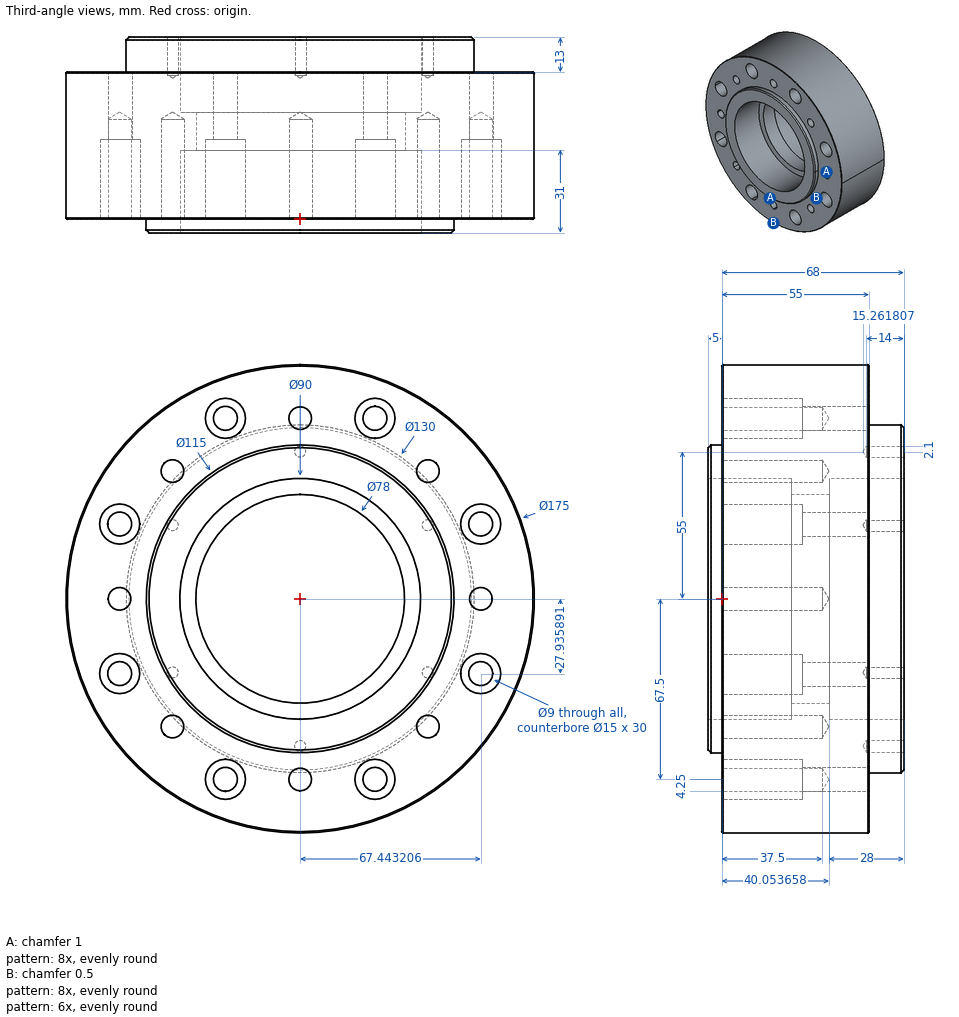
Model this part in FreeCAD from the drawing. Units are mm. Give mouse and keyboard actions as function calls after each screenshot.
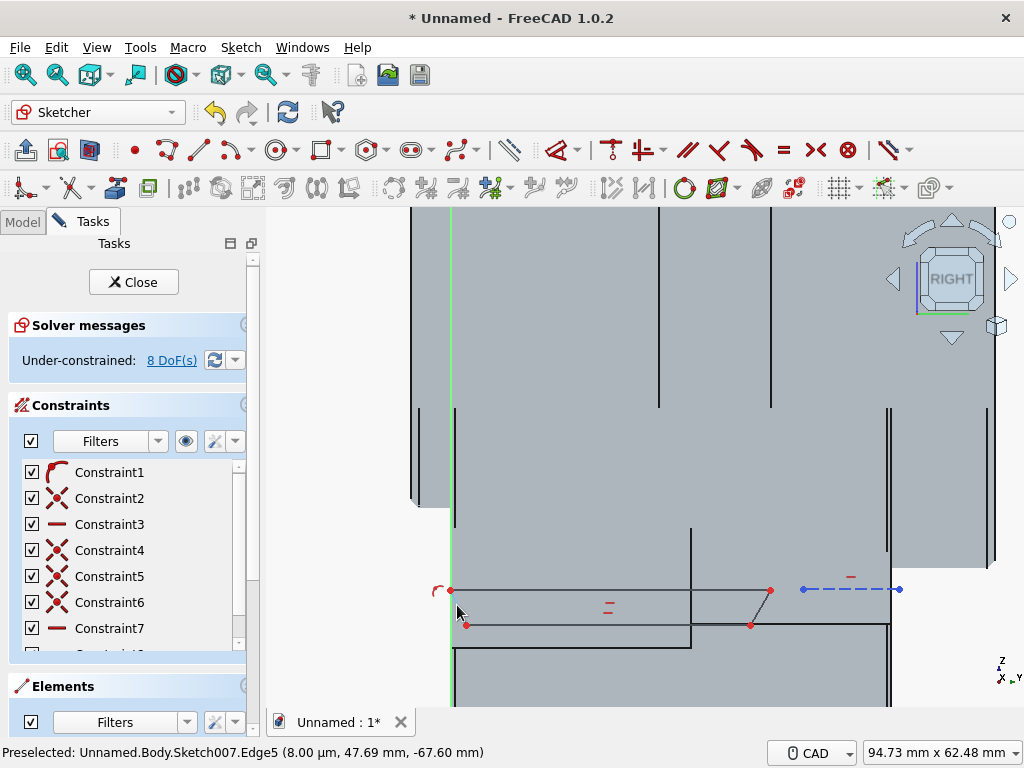
click(457, 604)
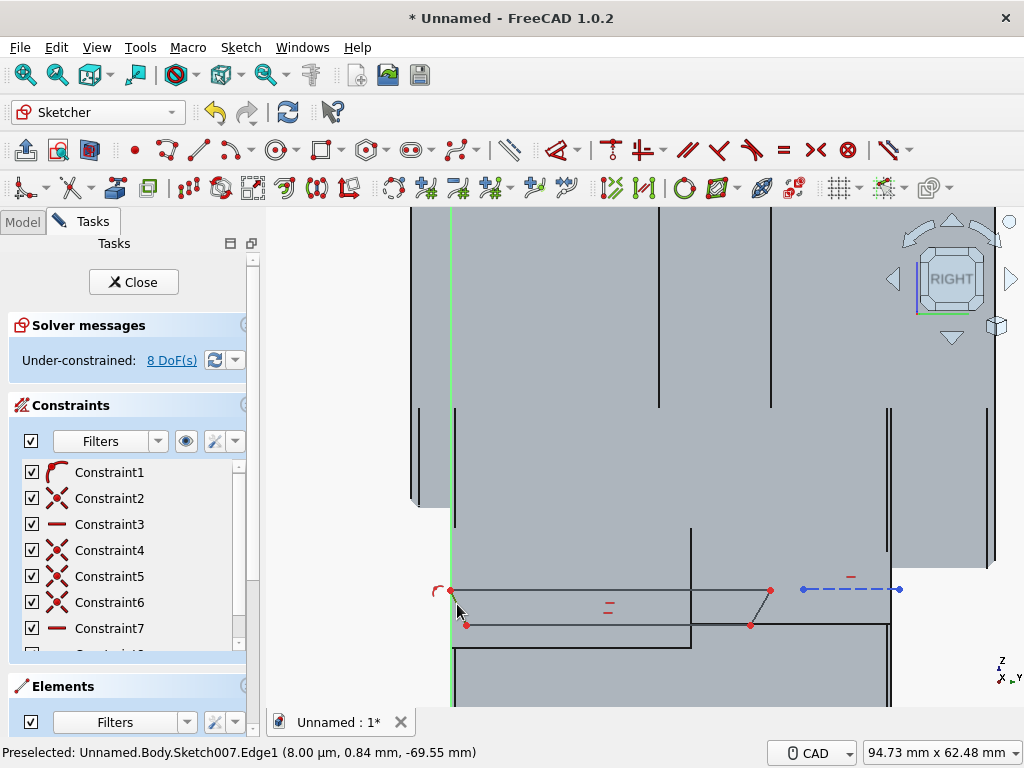
click(666, 150)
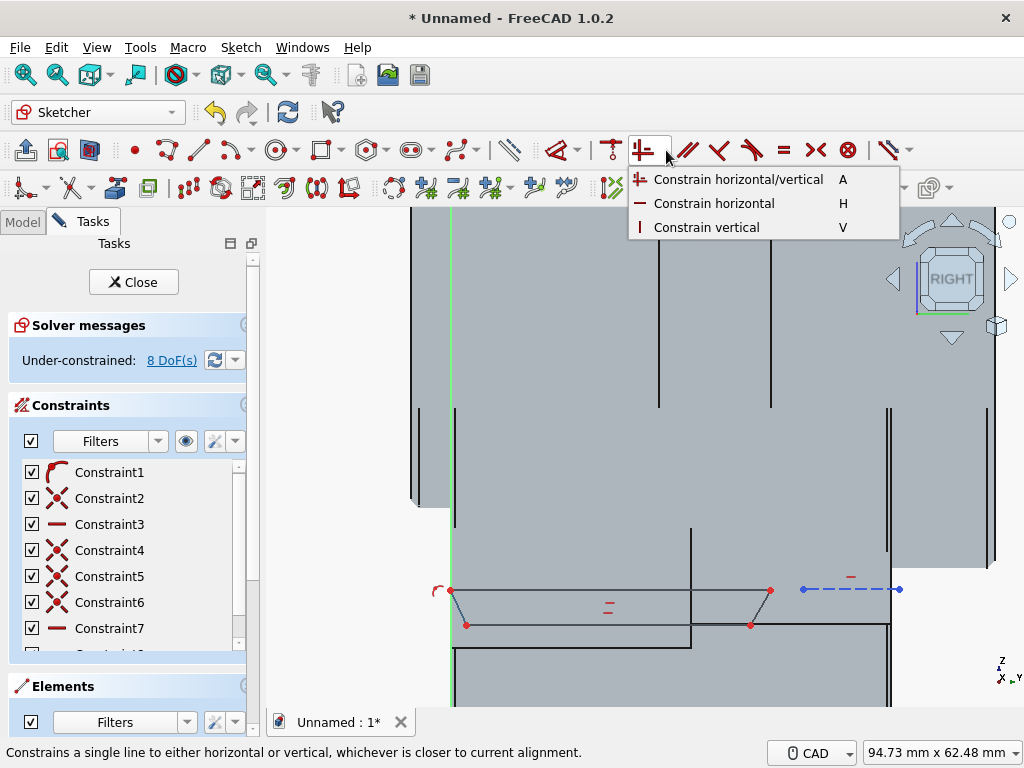
click(764, 227)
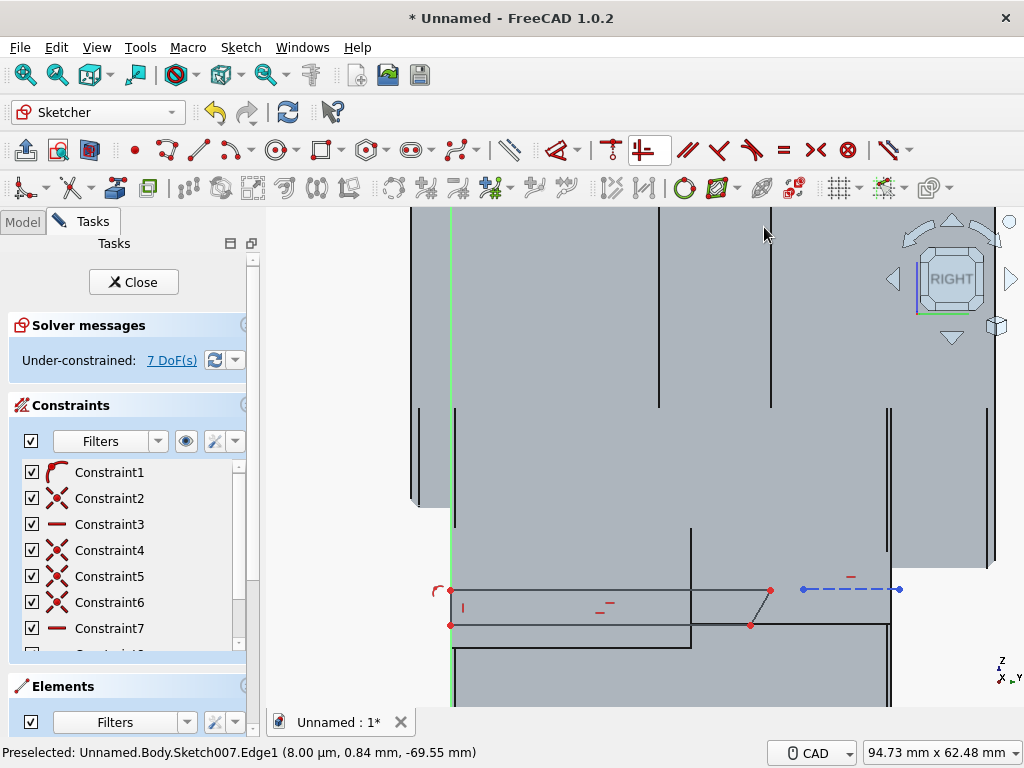
click(556, 150)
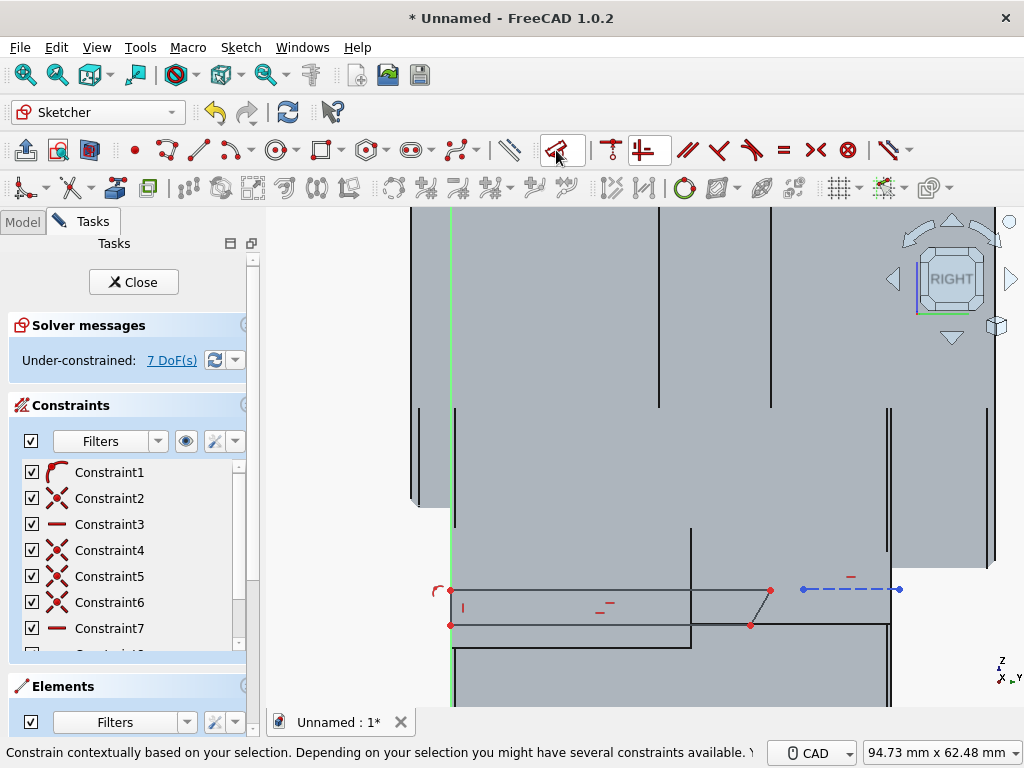
scroll(451, 601, up, 2)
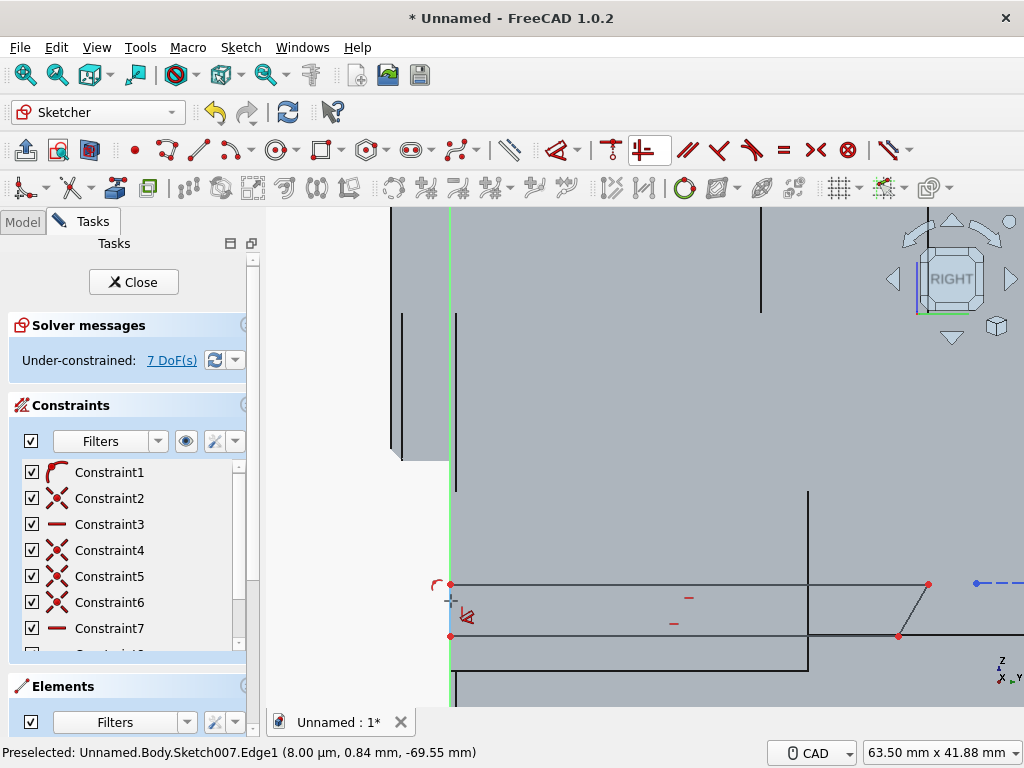
click(450, 600)
click(416, 611)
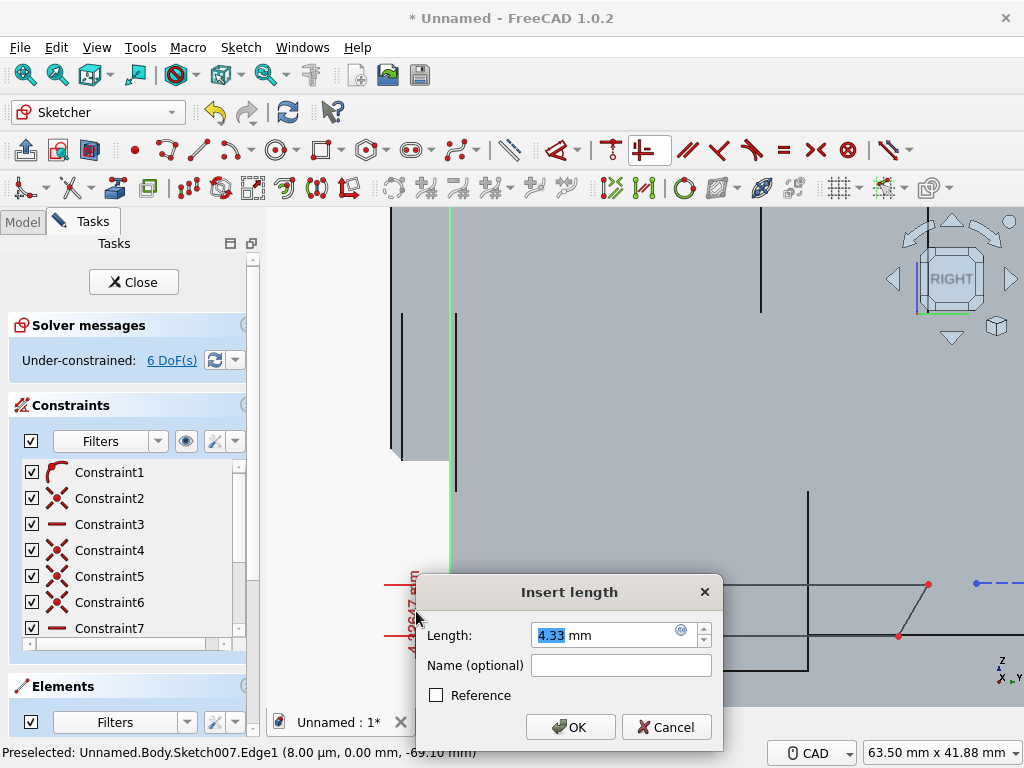
text(4.25)
key(Return)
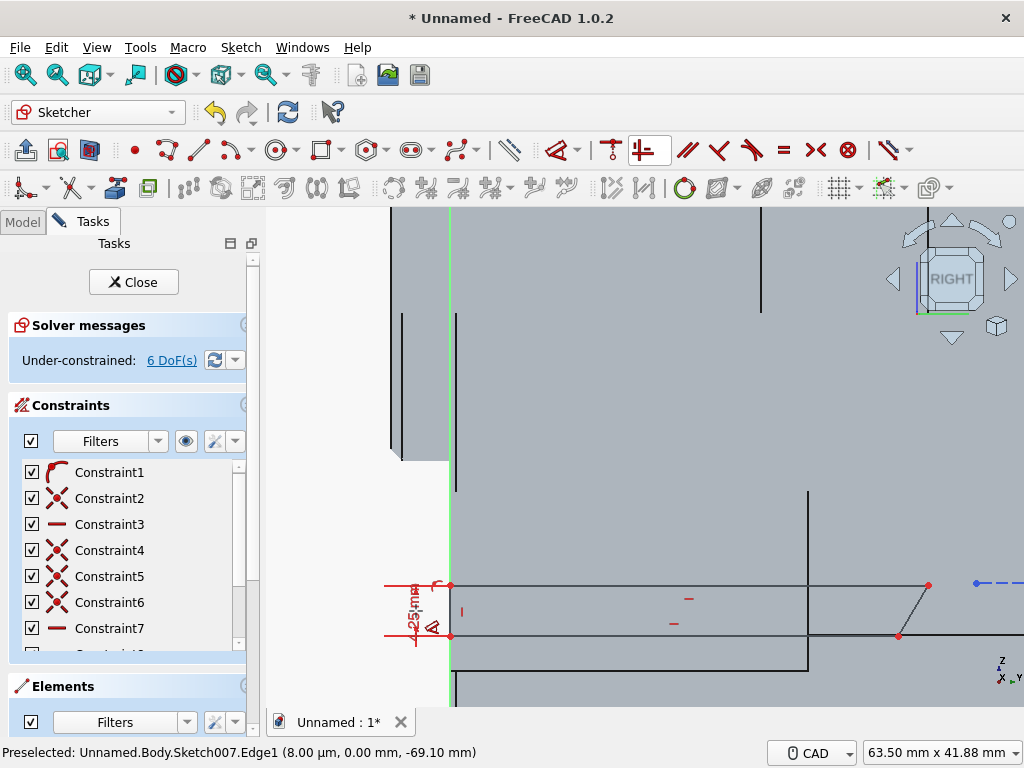
click(585, 636)
click(655, 670)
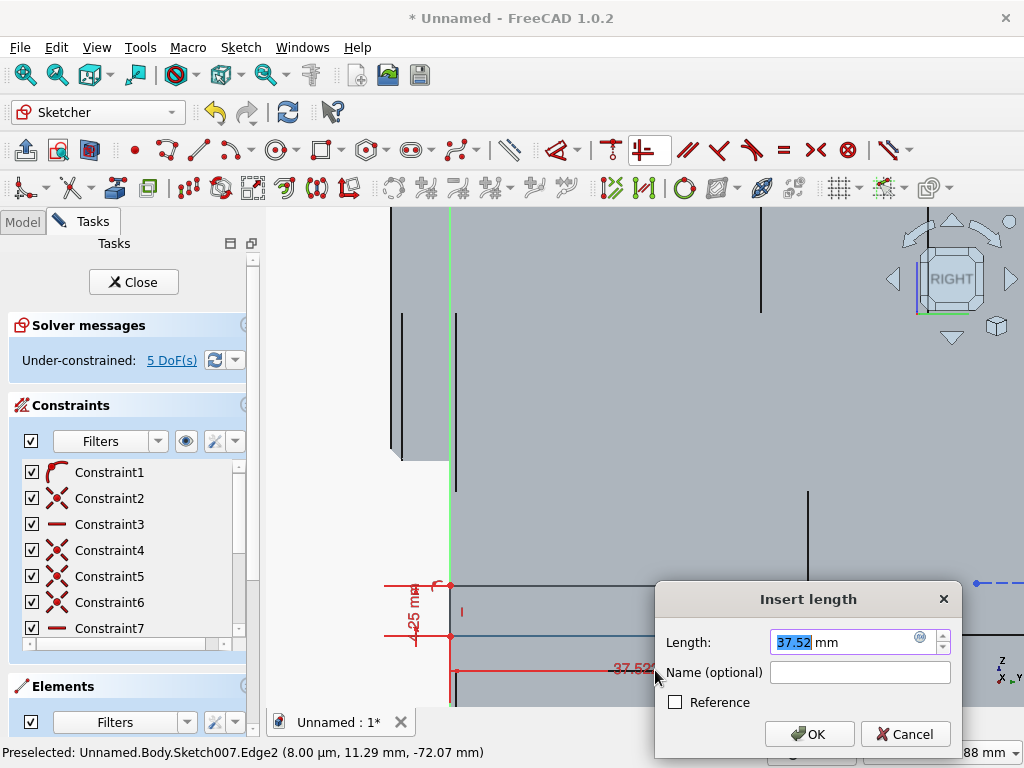
text(37.5)
key(Return)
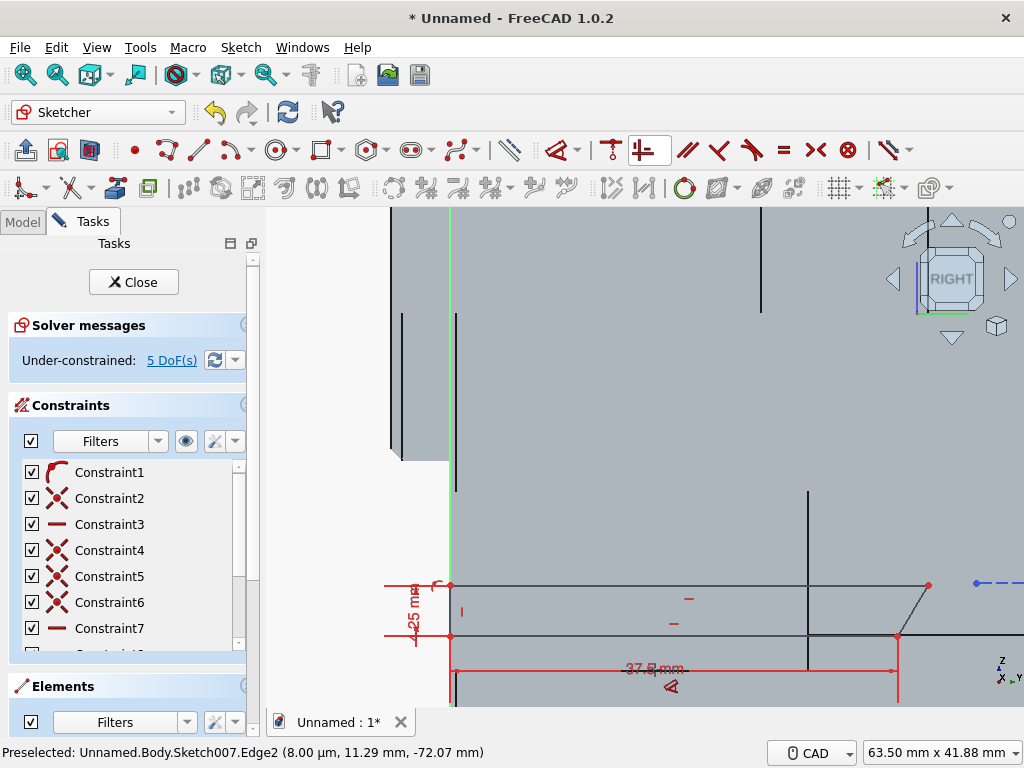
click(450, 586)
click(416, 410)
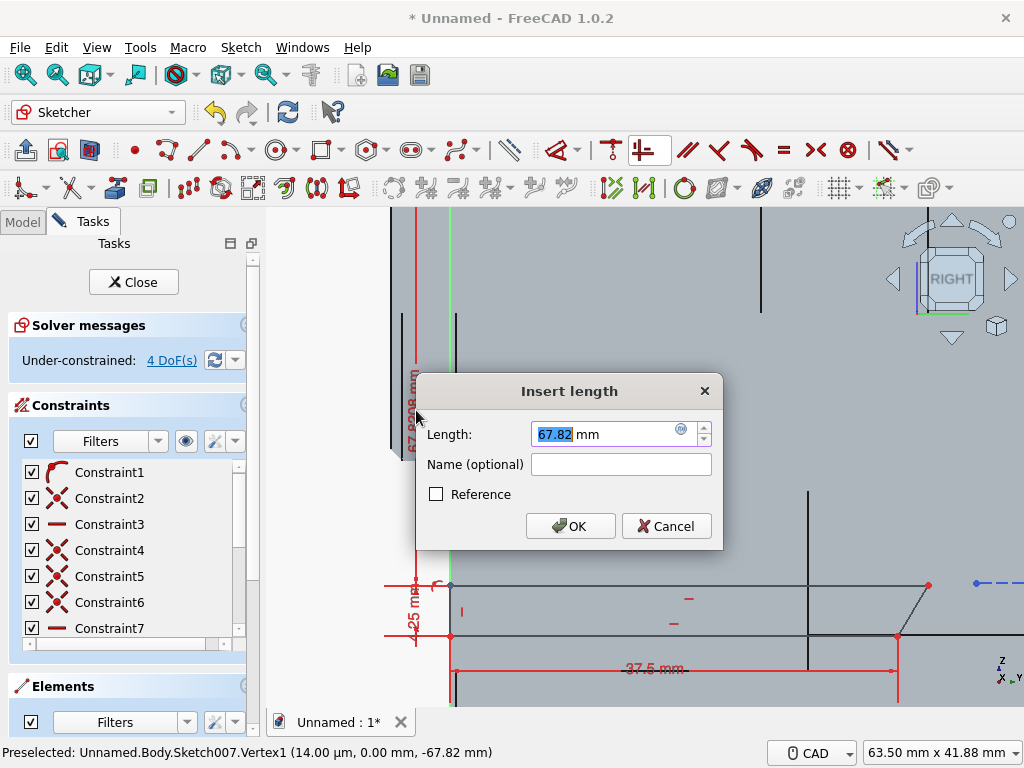
text(67.5)
key(Return)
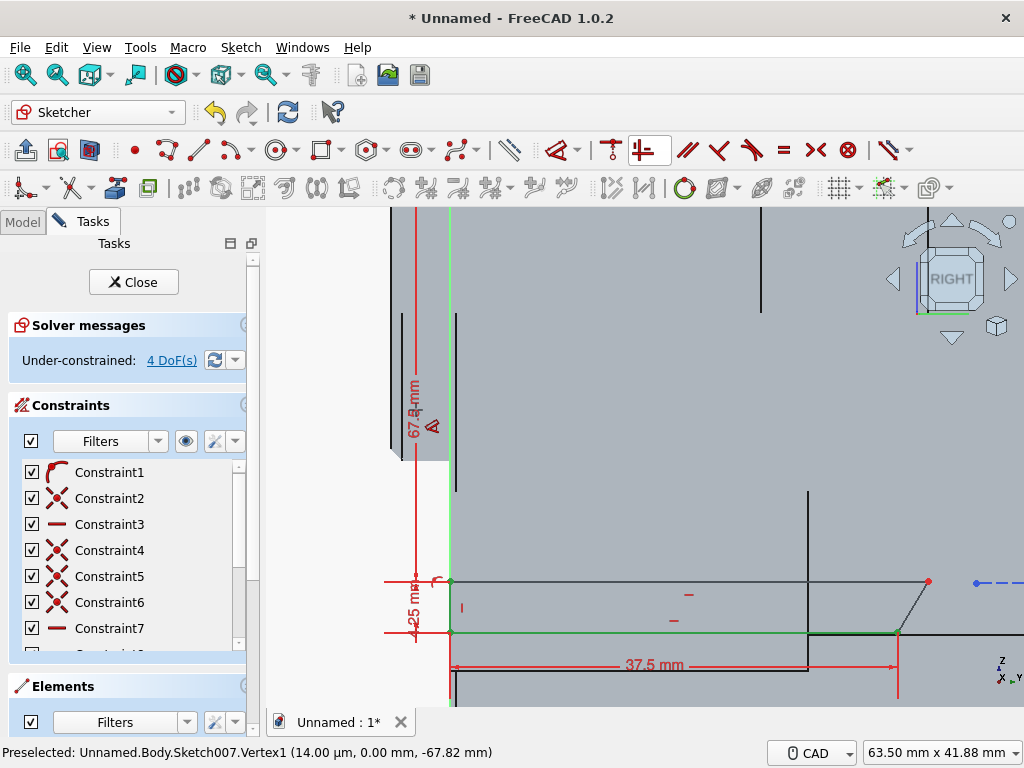
scroll(455, 604, down, 5)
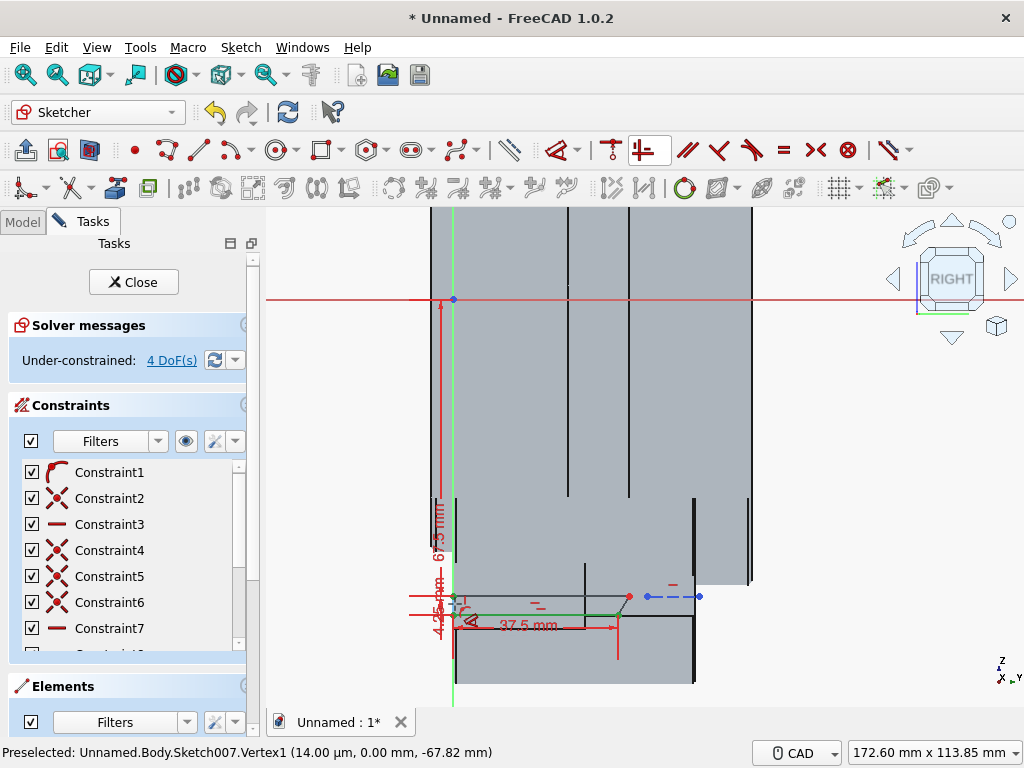
click(647, 597)
click(419, 448)